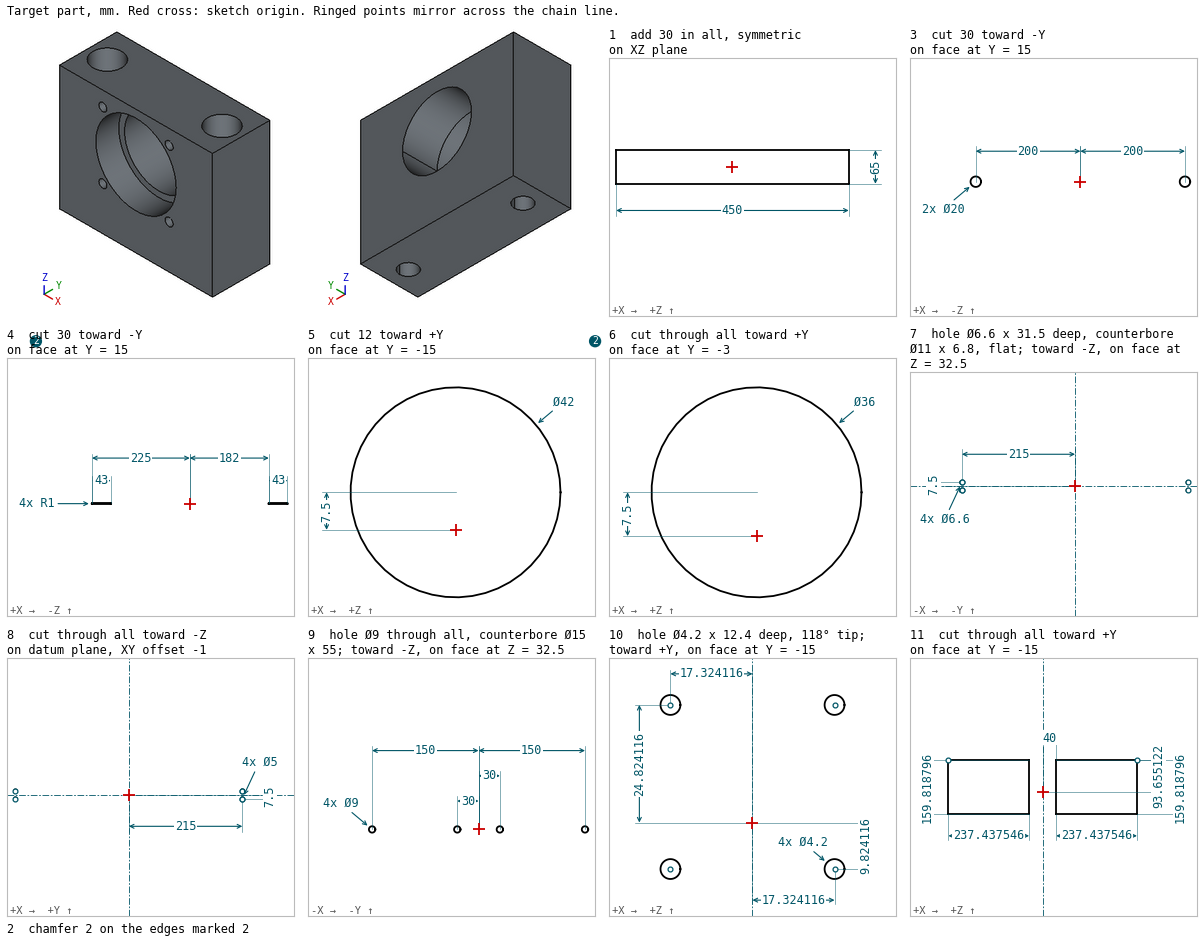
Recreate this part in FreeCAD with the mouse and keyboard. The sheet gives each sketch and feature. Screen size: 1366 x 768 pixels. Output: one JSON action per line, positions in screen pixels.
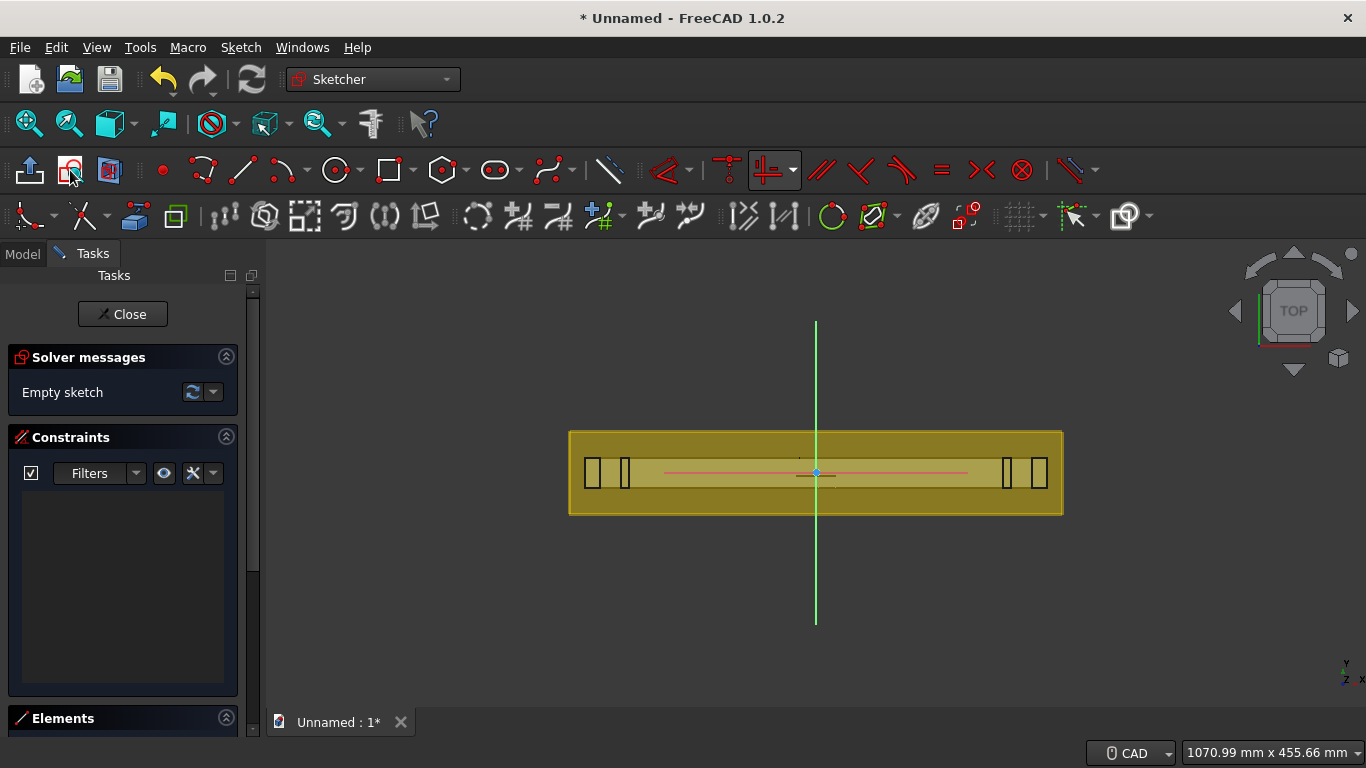
{"action": "scroll", "coordinate": [955, 473], "scroll_direction": "up", "scroll_amount": 2}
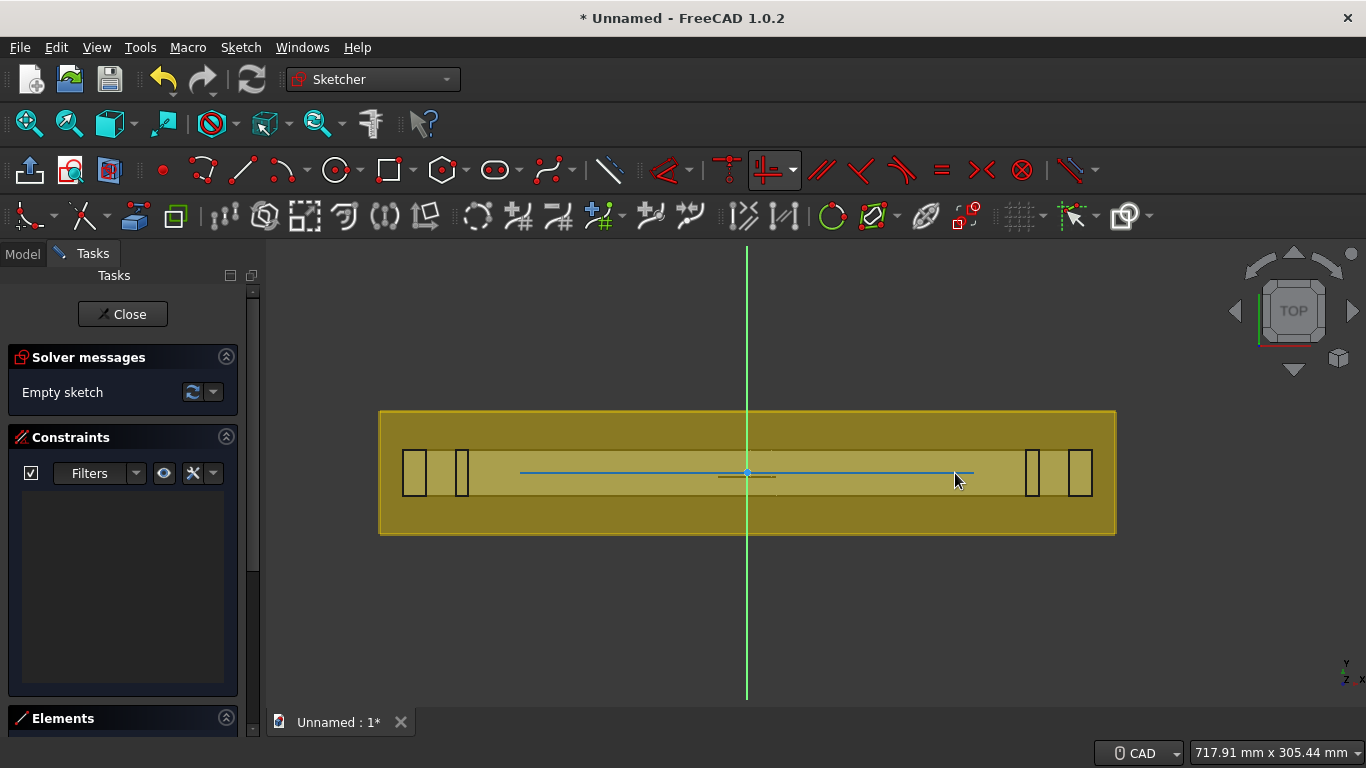
{"action": "key", "text": "g c"}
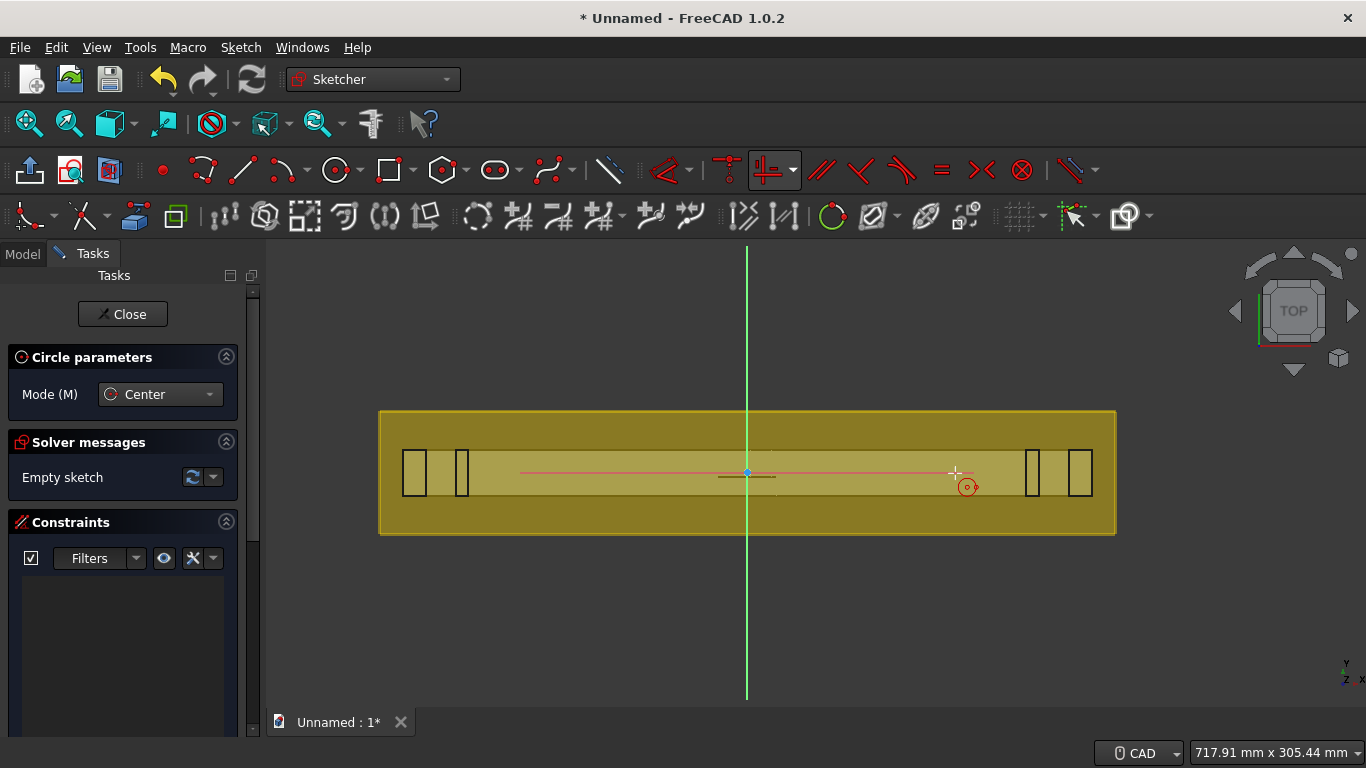
{"action": "scroll", "coordinate": [1077, 484], "scroll_direction": "up", "scroll_amount": 9}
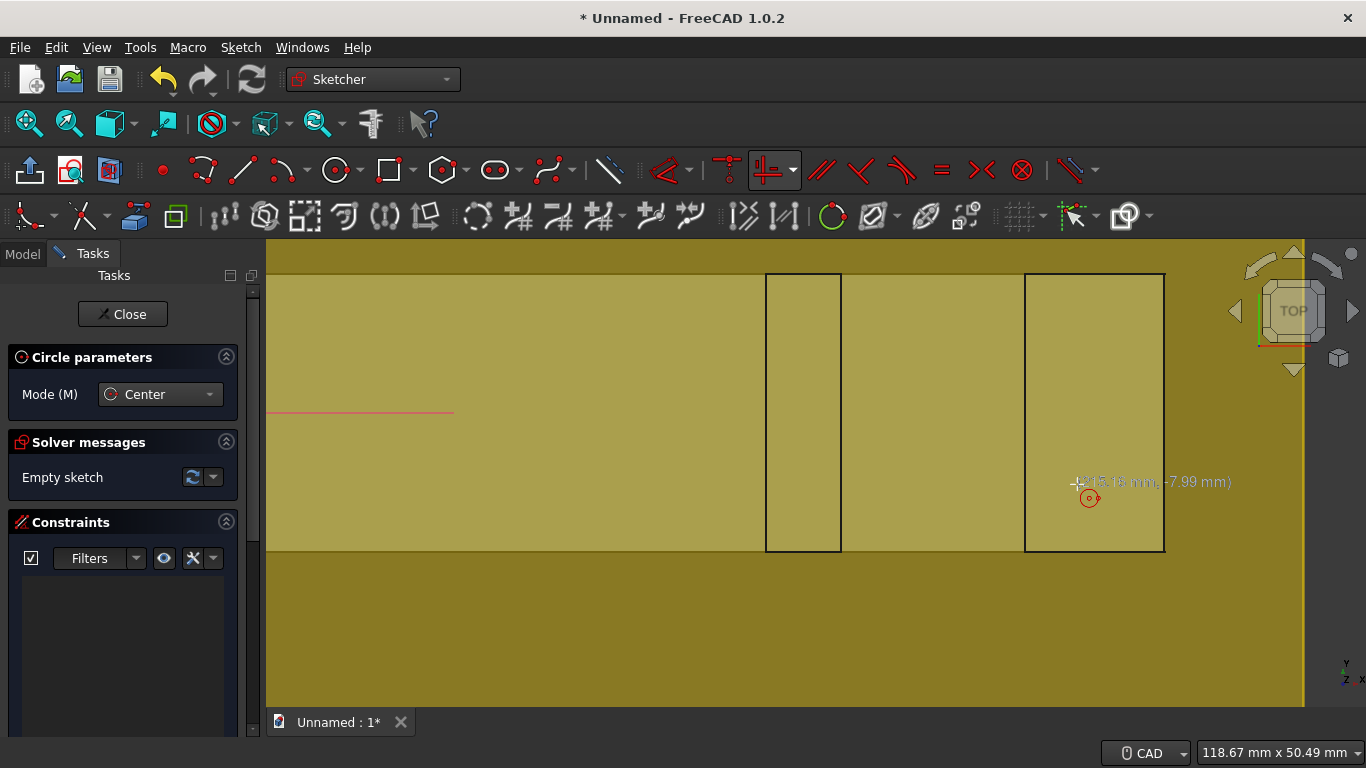
{"action": "scroll", "coordinate": [1078, 485], "scroll_direction": "down", "scroll_amount": 9}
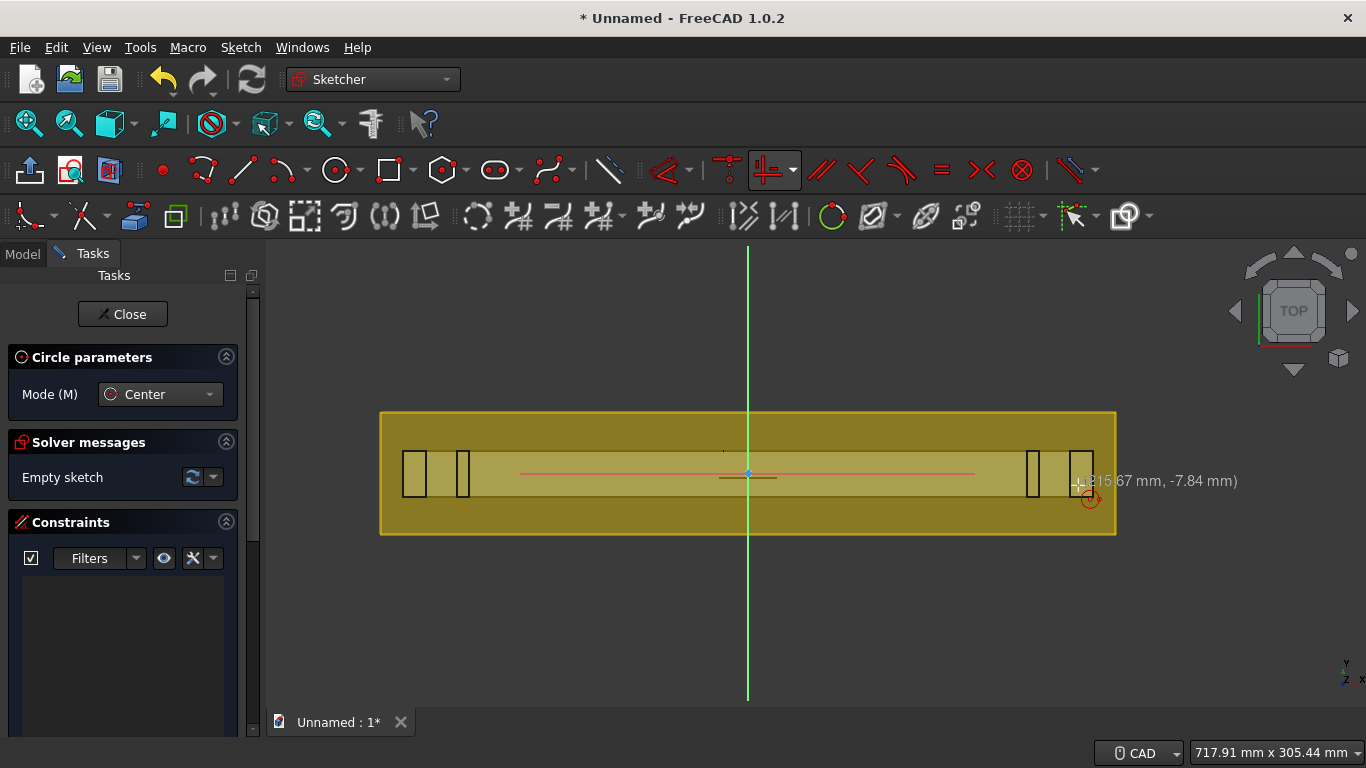
{"action": "scroll", "coordinate": [1078, 485], "scroll_direction": "up", "scroll_amount": 2}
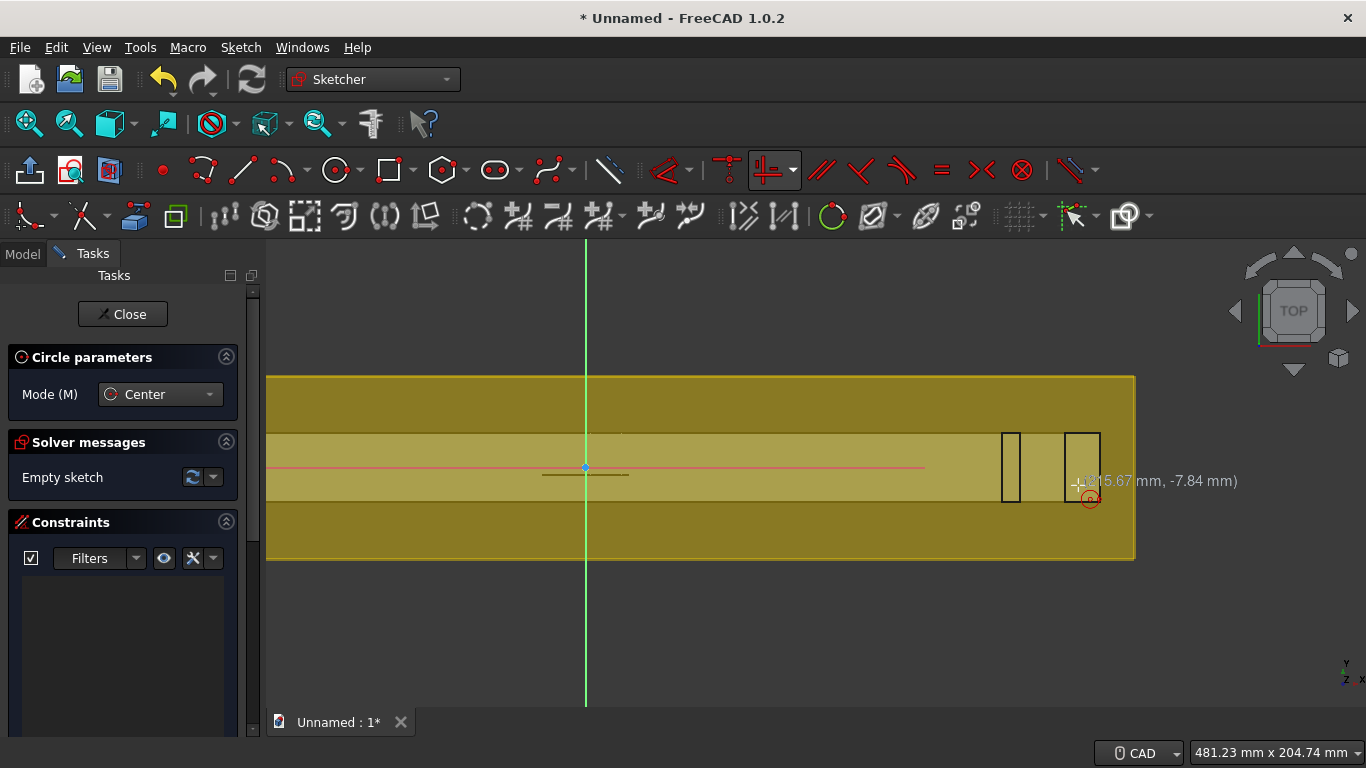
{"action": "left_click", "coordinate": [1077, 485]}
{"action": "mouse_move", "coordinate": [1081, 489]}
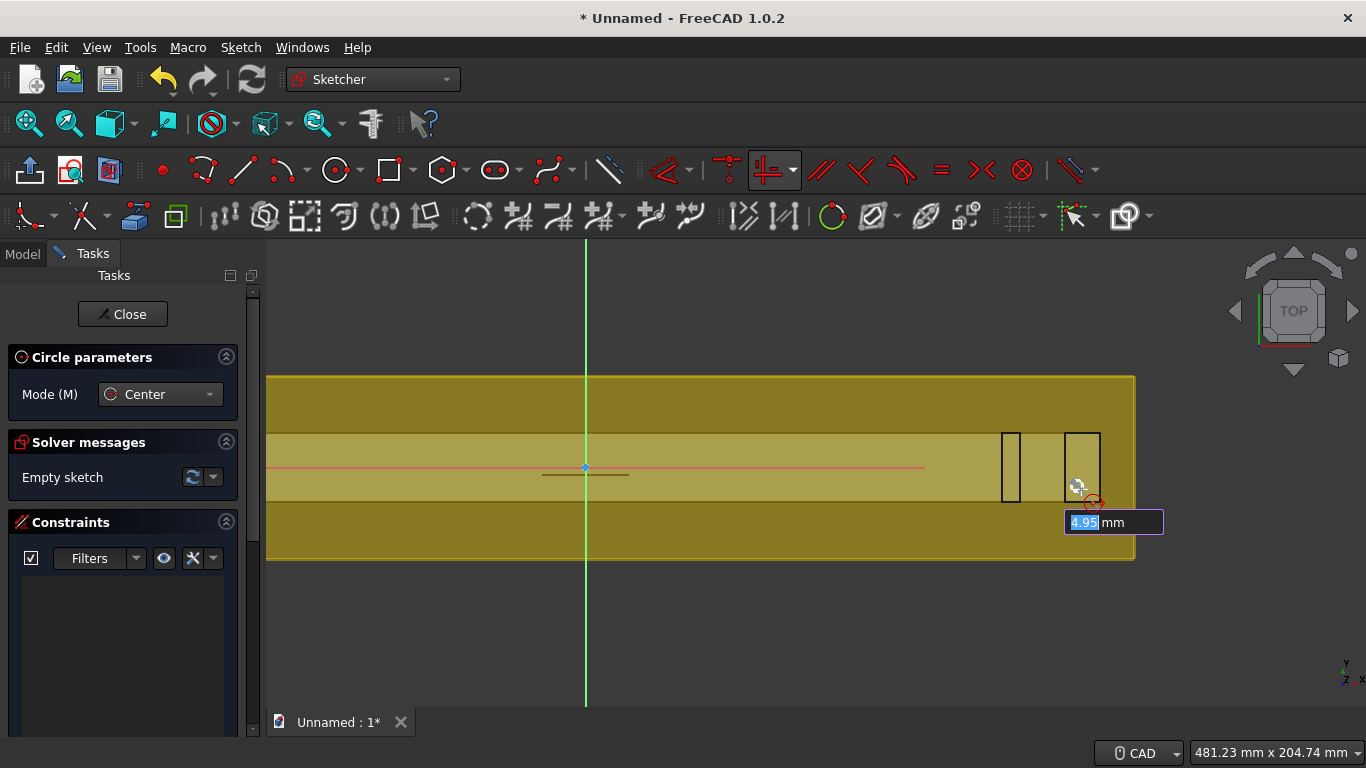
{"action": "type", "text": "5"}
{"action": "key", "text": "Return"}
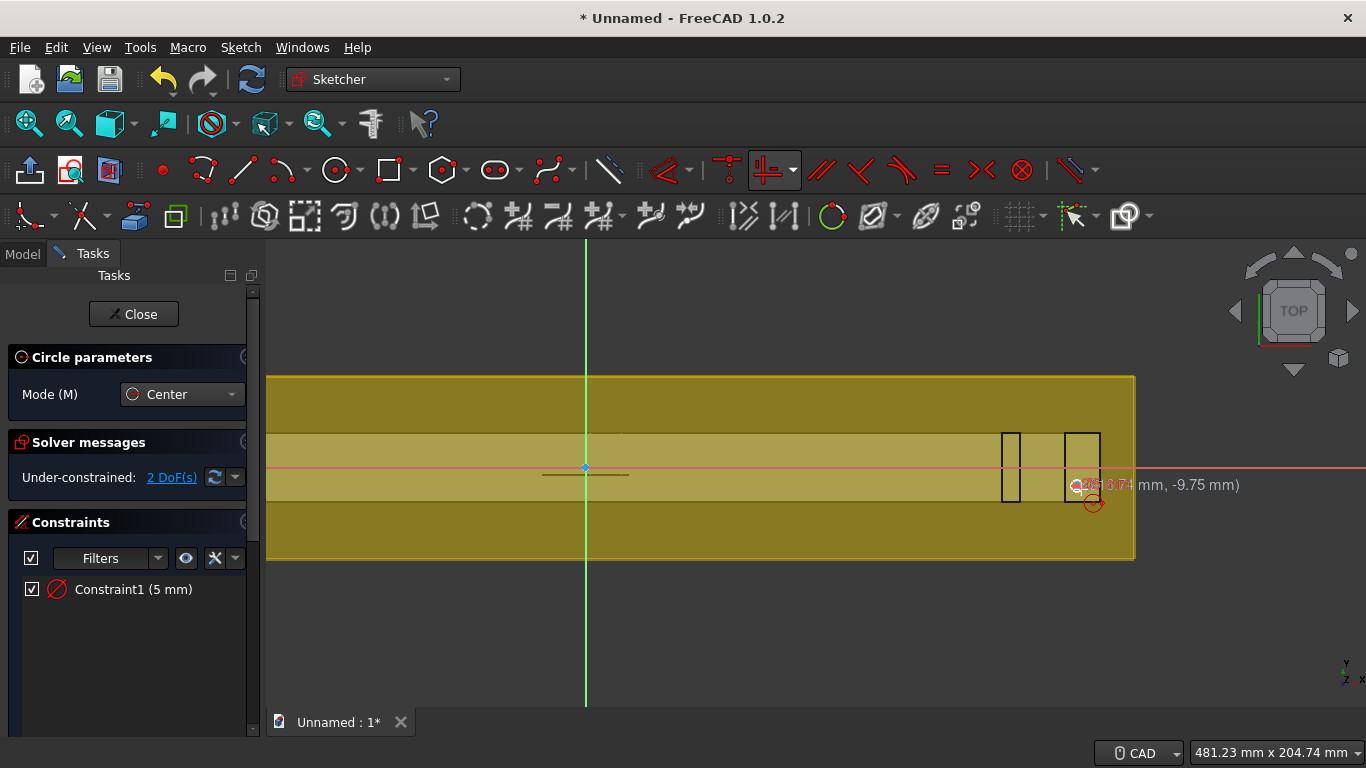
{"action": "scroll", "coordinate": [1077, 451], "scroll_direction": "up", "scroll_amount": 7}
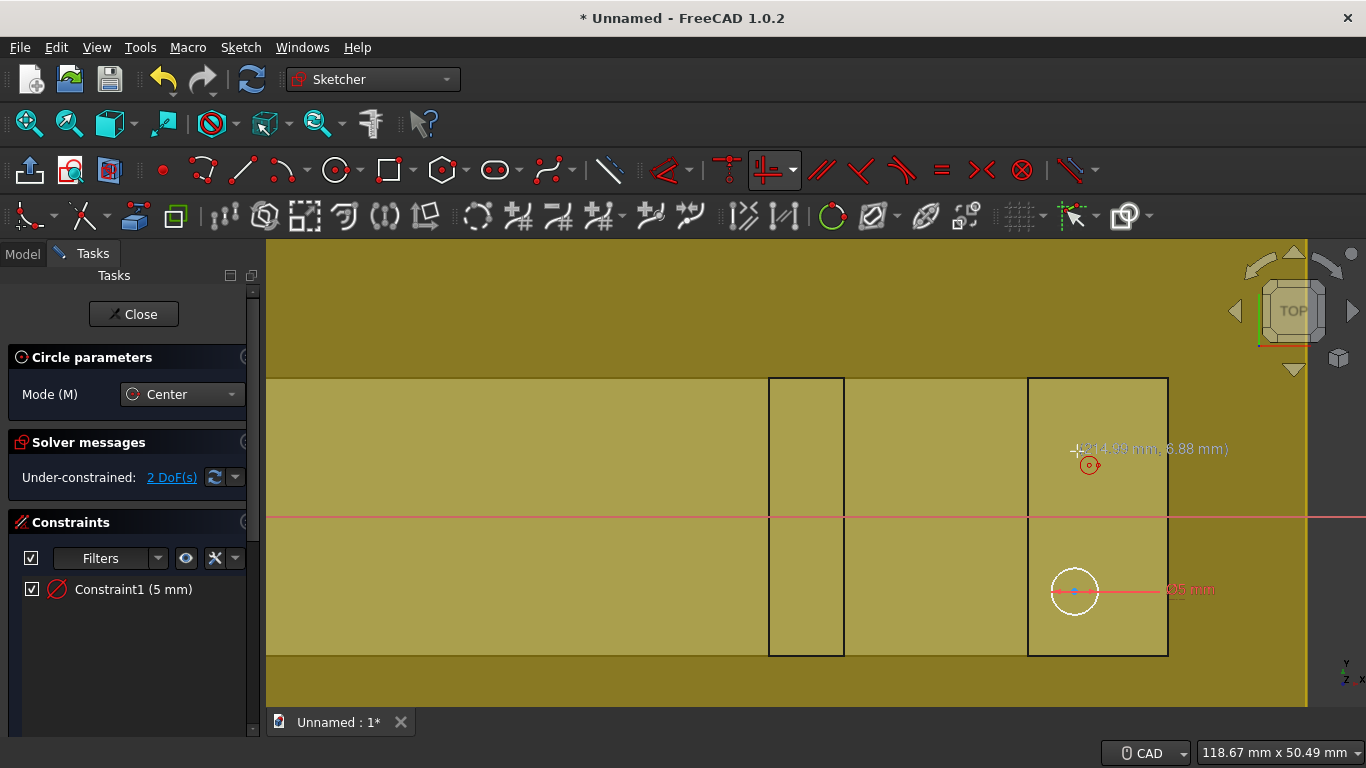
{"action": "scroll", "coordinate": [1077, 464], "scroll_direction": "down", "scroll_amount": 9}